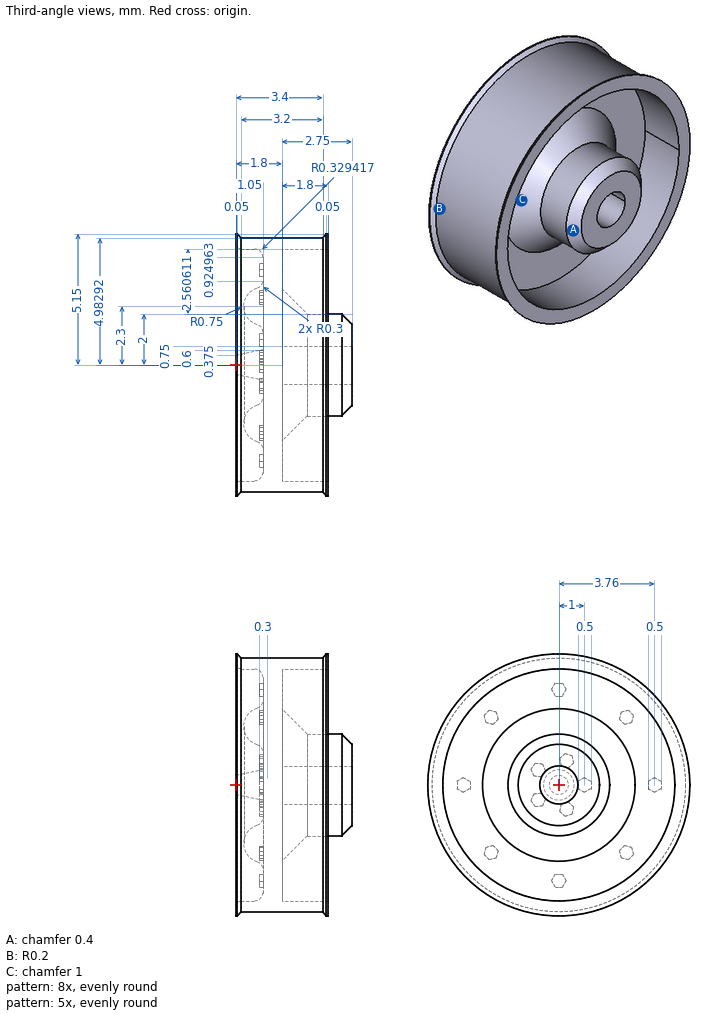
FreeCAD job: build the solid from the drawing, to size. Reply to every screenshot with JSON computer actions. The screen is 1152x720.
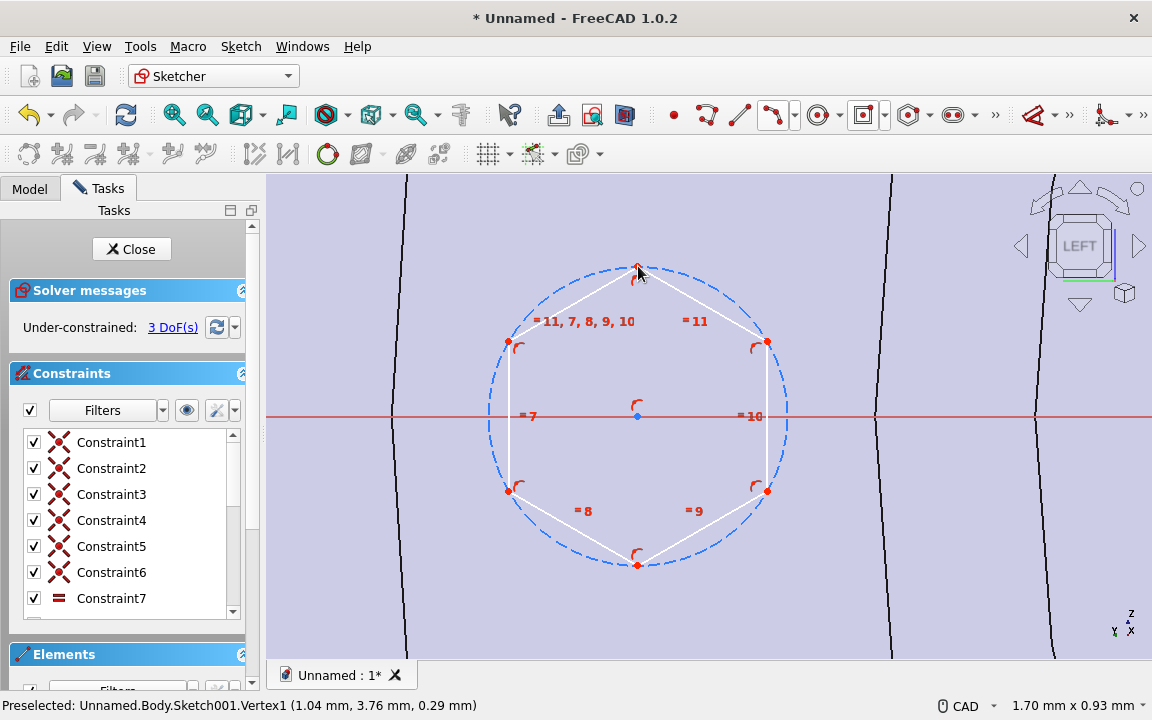
{"action": "left_click", "coordinate": [509, 387]}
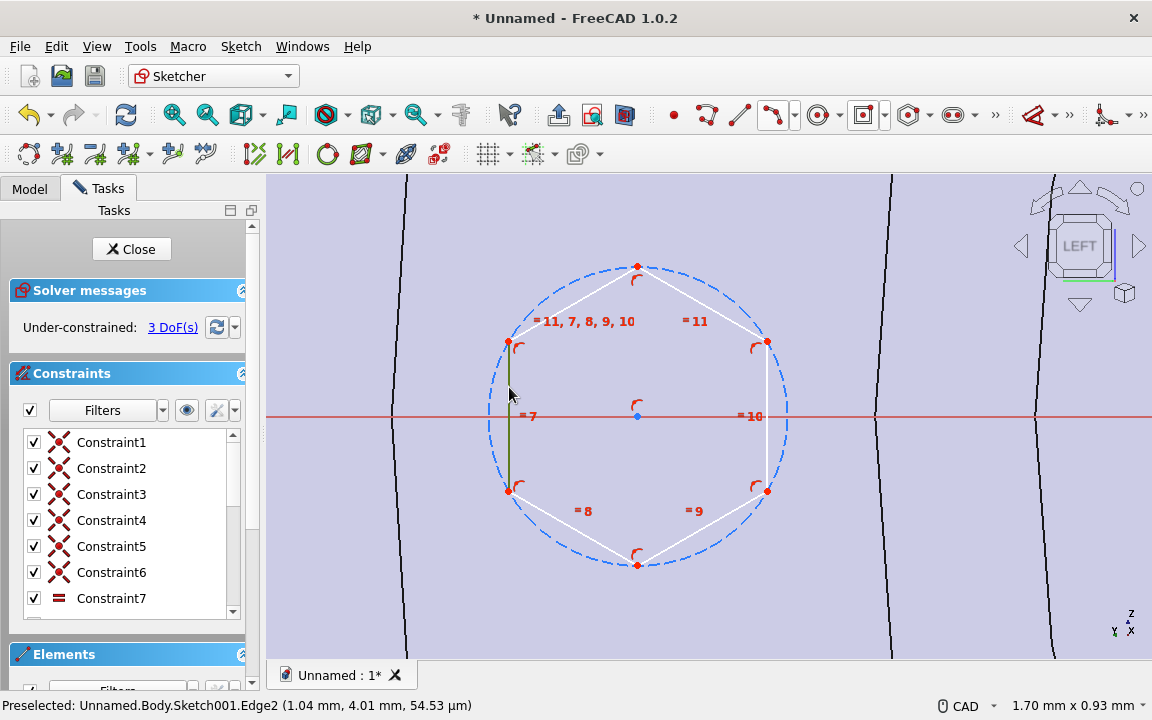
{"action": "key", "text": "v"}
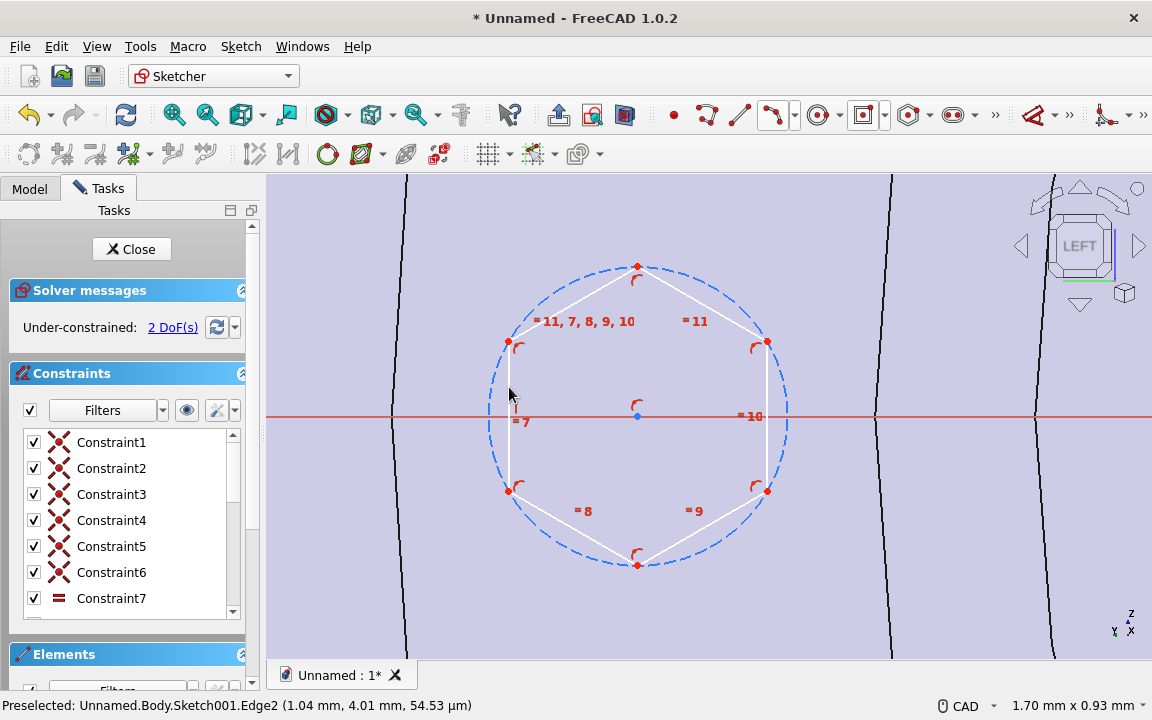
{"action": "left_click", "coordinate": [1032, 116]}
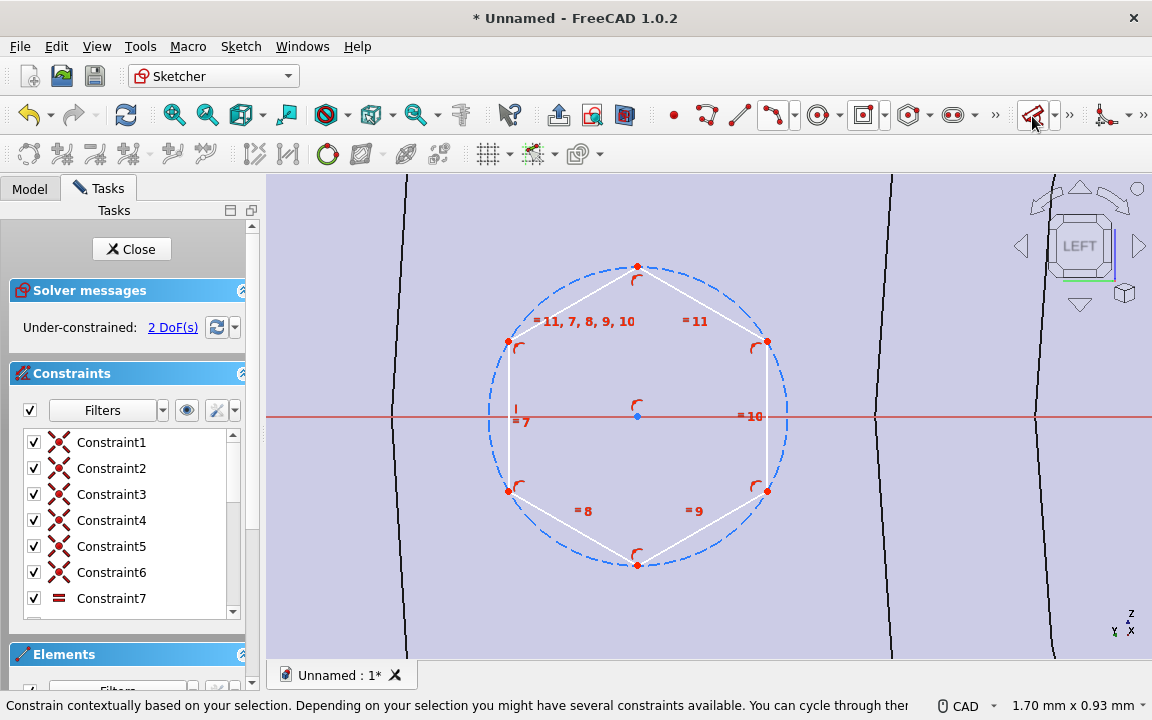
{"action": "left_click", "coordinate": [509, 342]}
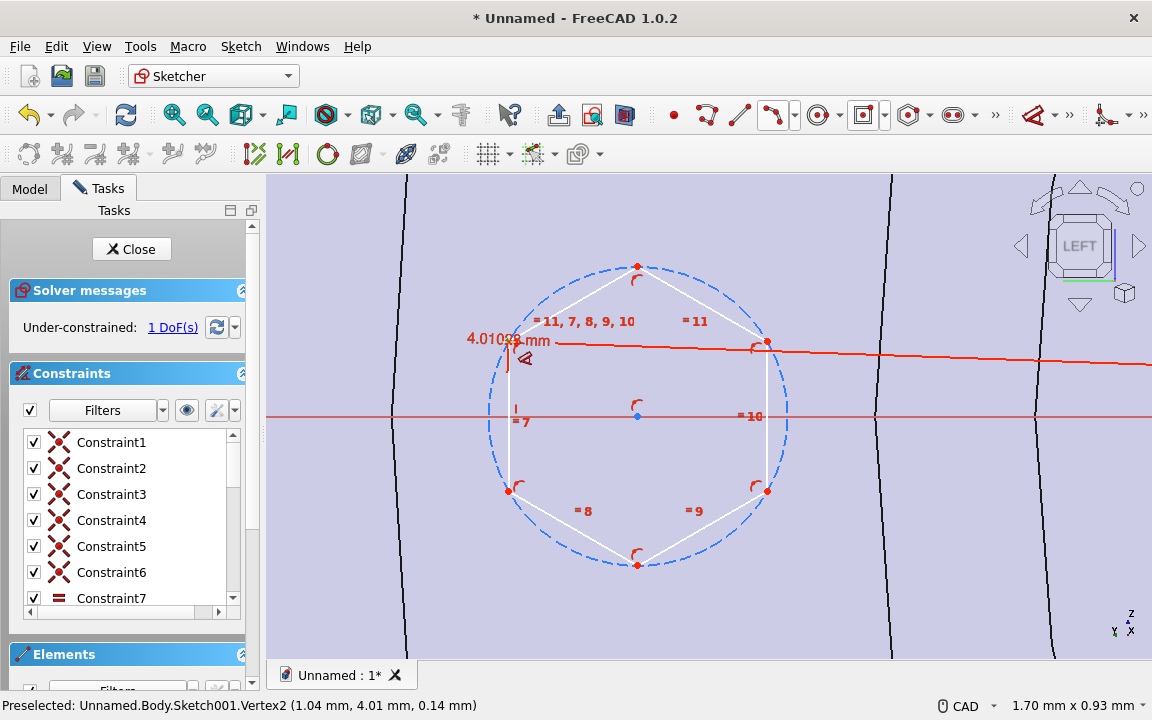
{"action": "left_click", "coordinate": [767, 491]}
{"action": "left_click", "coordinate": [638, 525]}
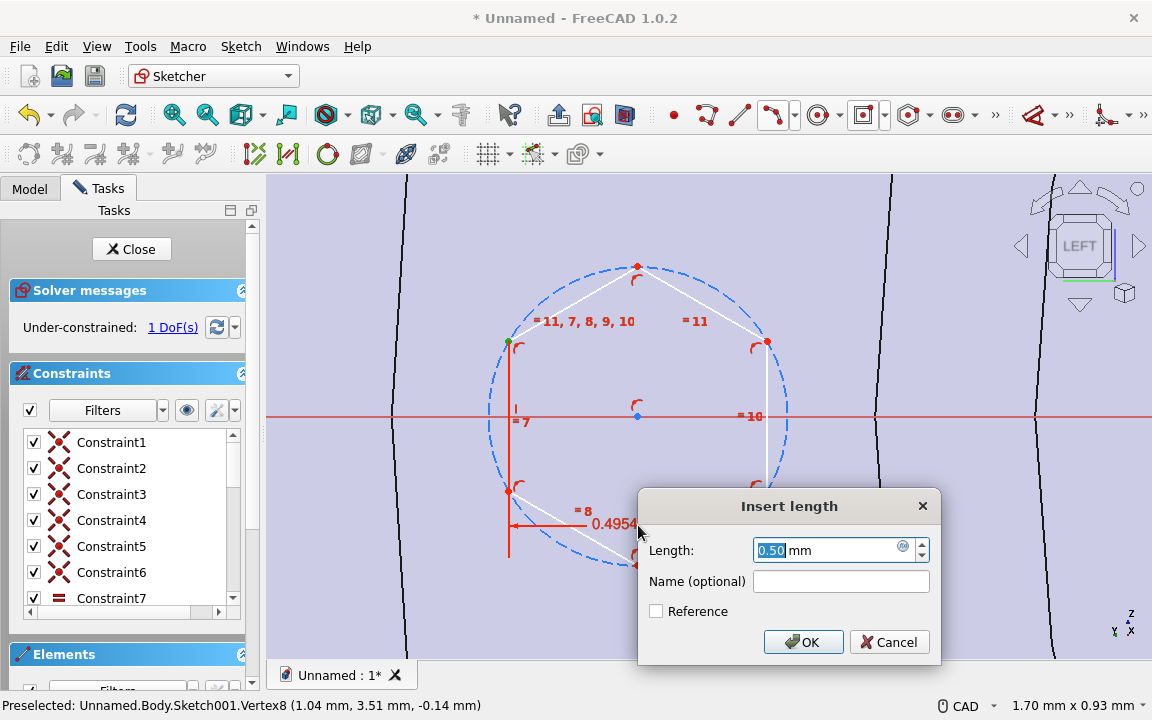
{"action": "type", "text": "0.5"}
{"action": "key", "text": "Return"}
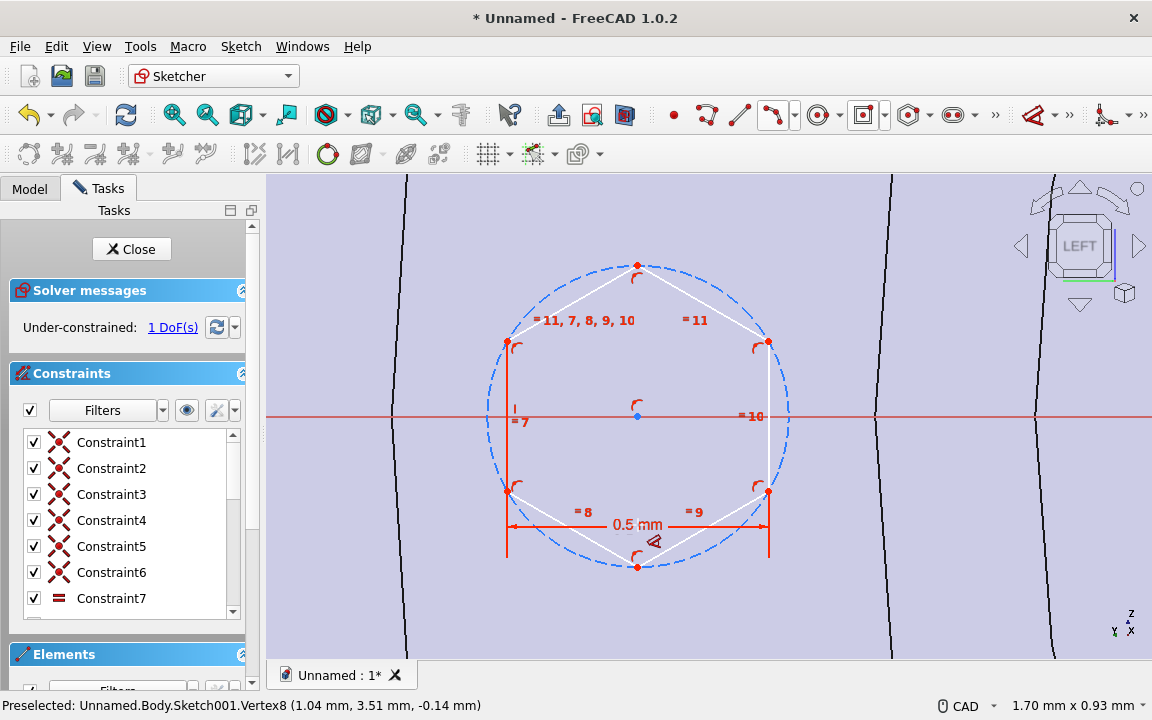
{"action": "left_click", "coordinate": [638, 416]}
{"action": "left_click", "coordinate": [812, 450]}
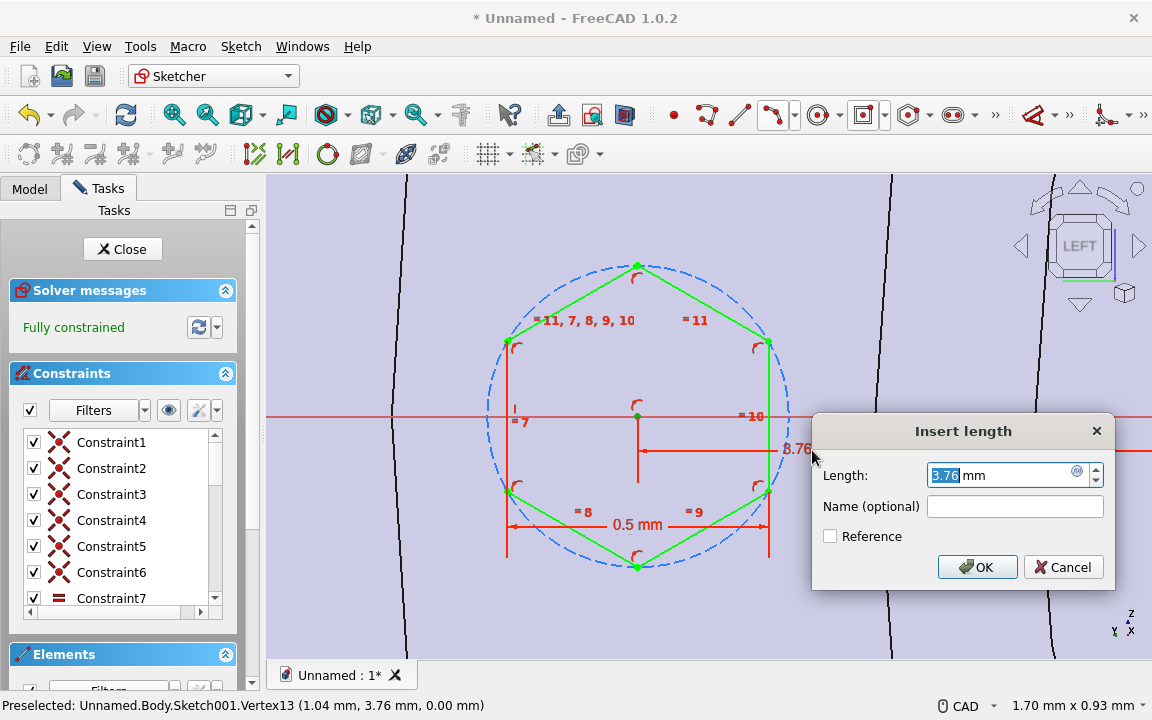
{"action": "type", "text": "3.76"}
{"action": "key", "text": "Return"}
{"action": "key", "text": "Escape"}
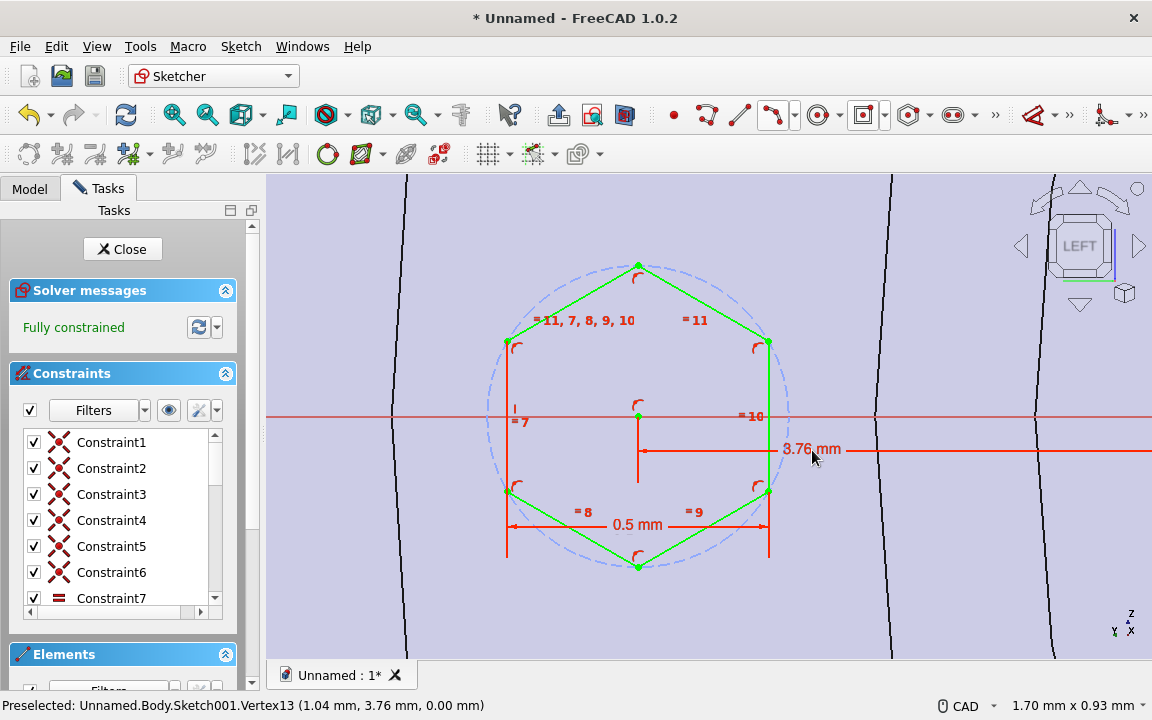
{"action": "left_click", "coordinate": [123, 249]}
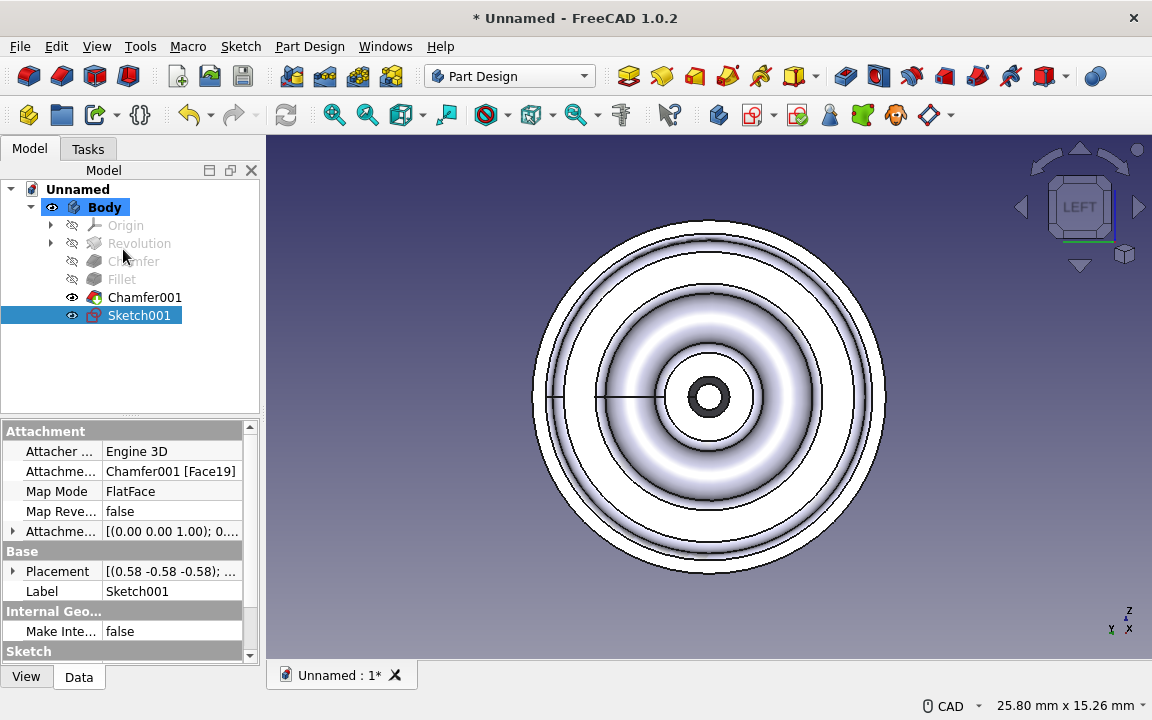
{"action": "left_click", "coordinate": [629, 76]}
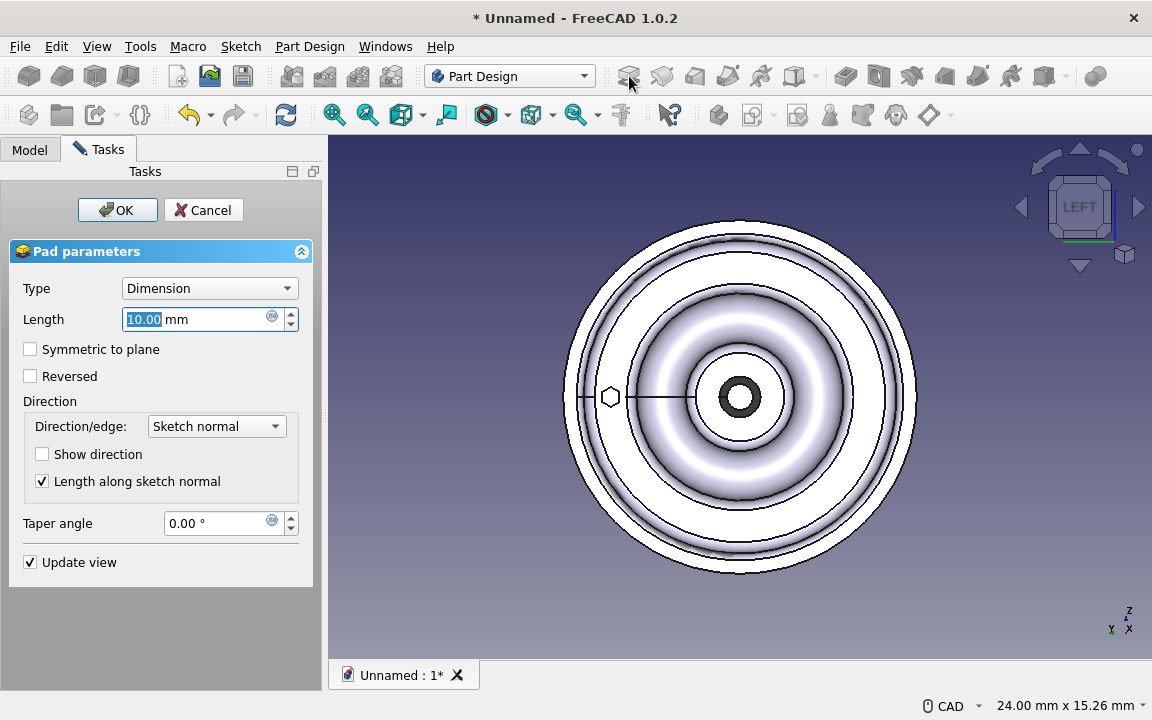
{"action": "type", "text": "0.3"}
{"action": "key", "text": "Tab"}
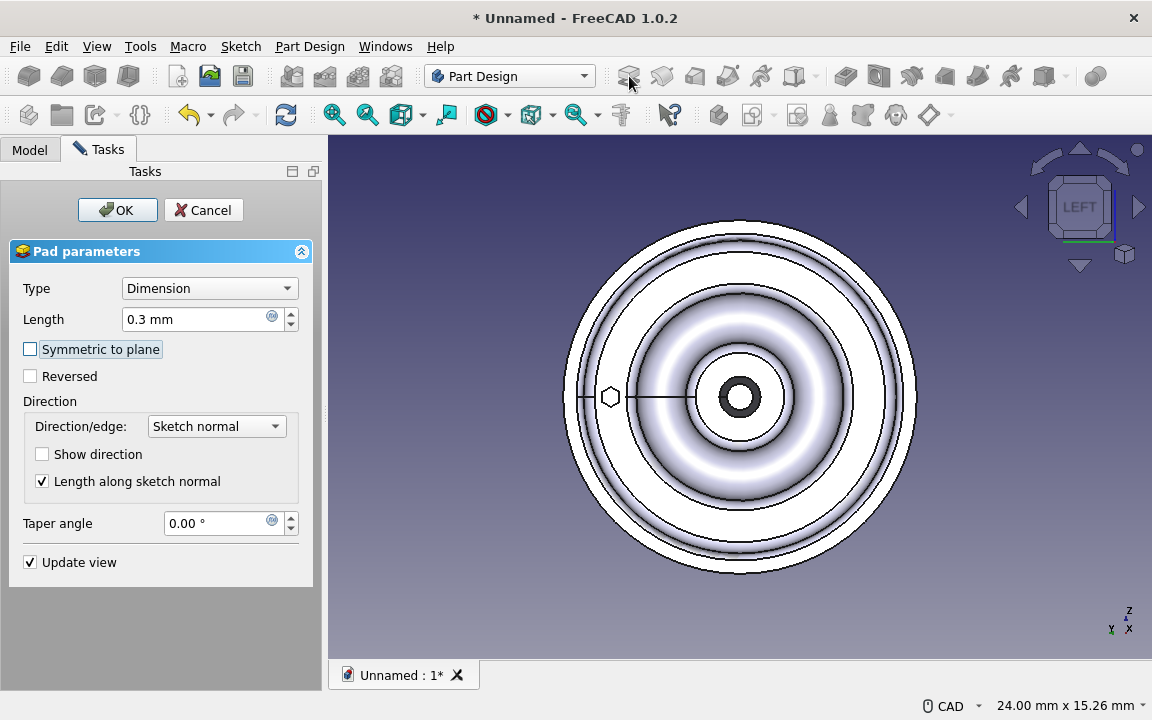
{"action": "left_click", "coordinate": [31, 349]}